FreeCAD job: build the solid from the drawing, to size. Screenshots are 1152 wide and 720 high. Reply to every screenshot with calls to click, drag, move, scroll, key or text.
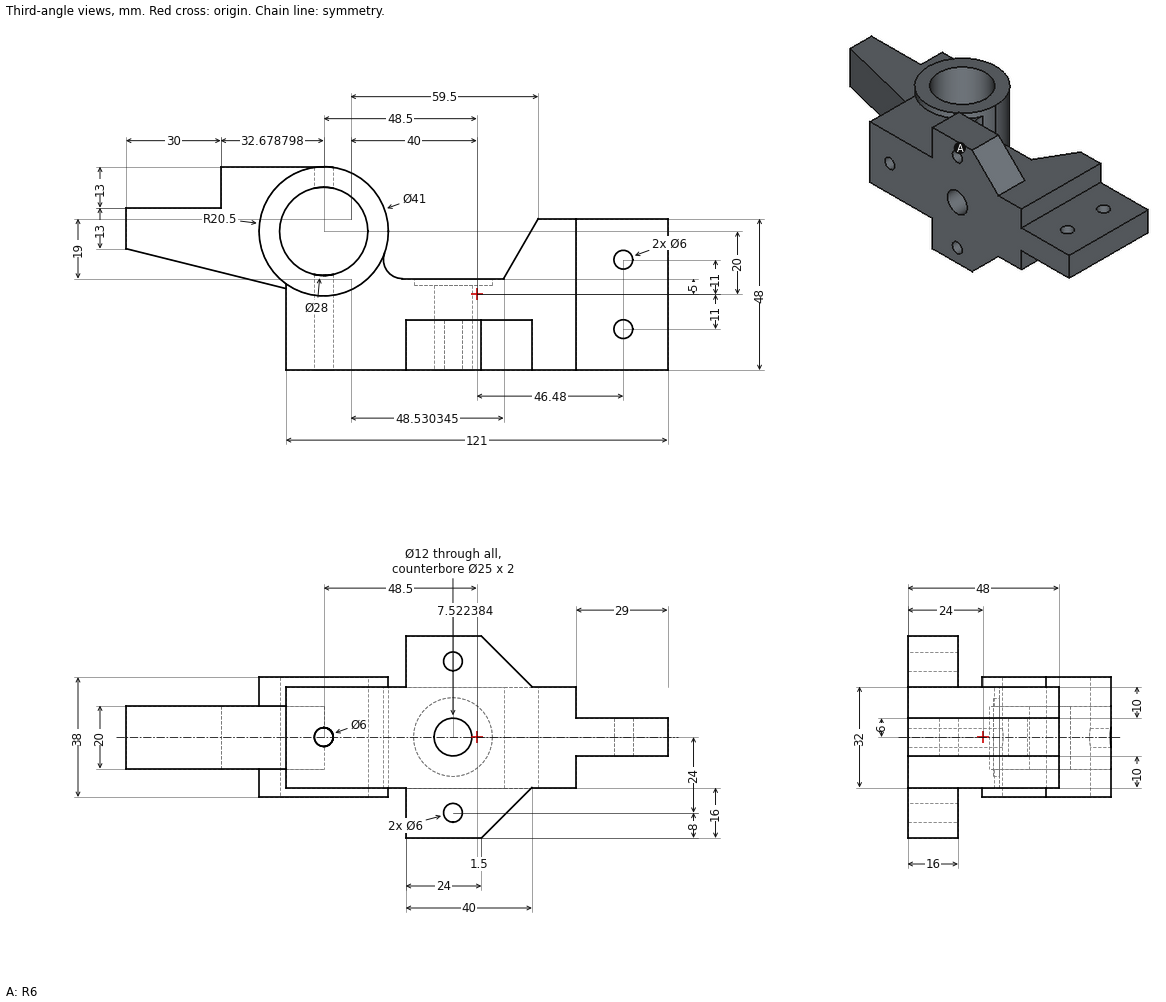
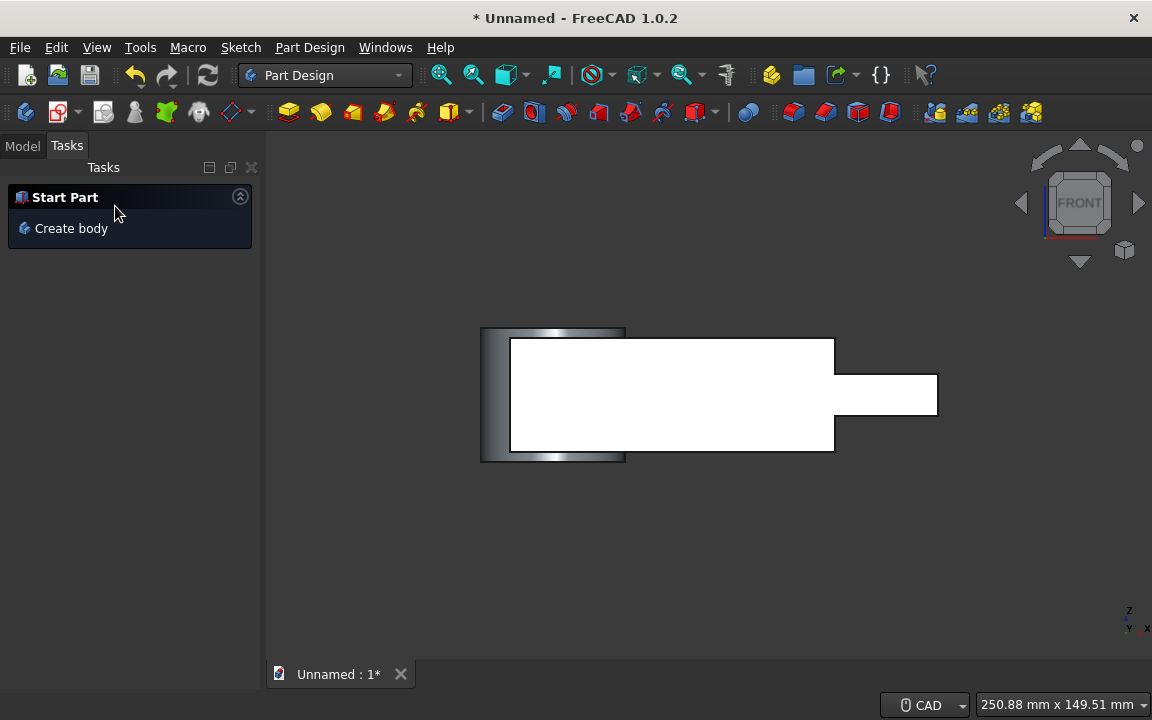
key(3)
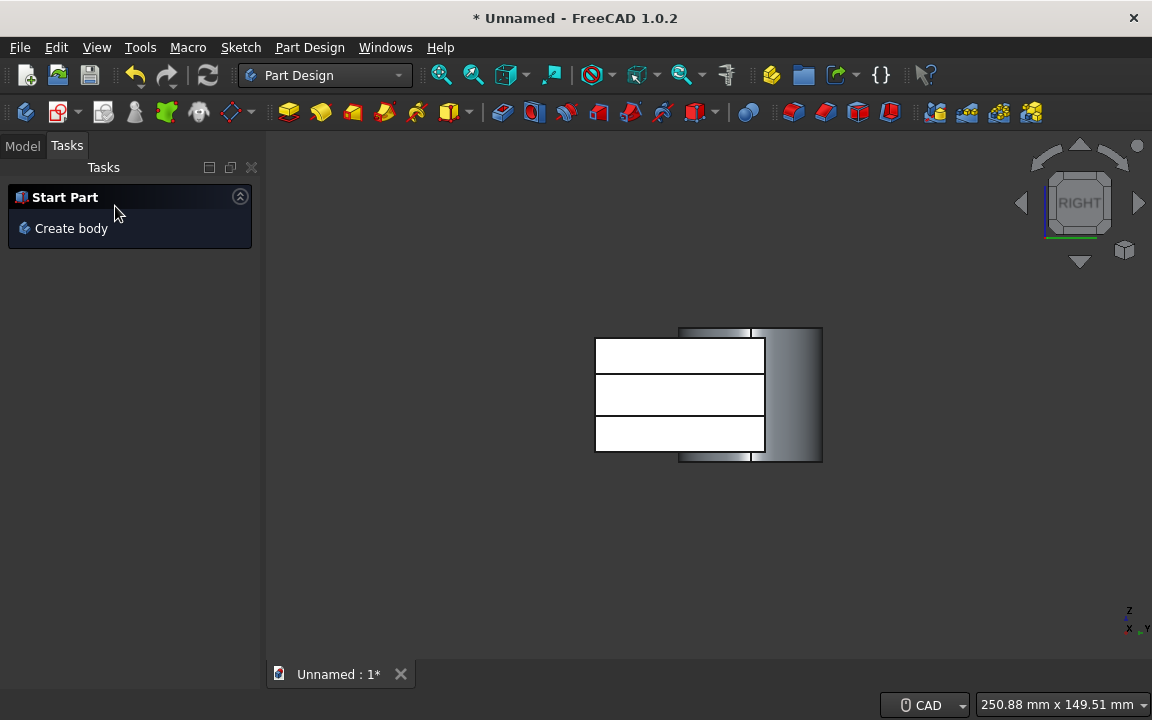
key(v)
key(f)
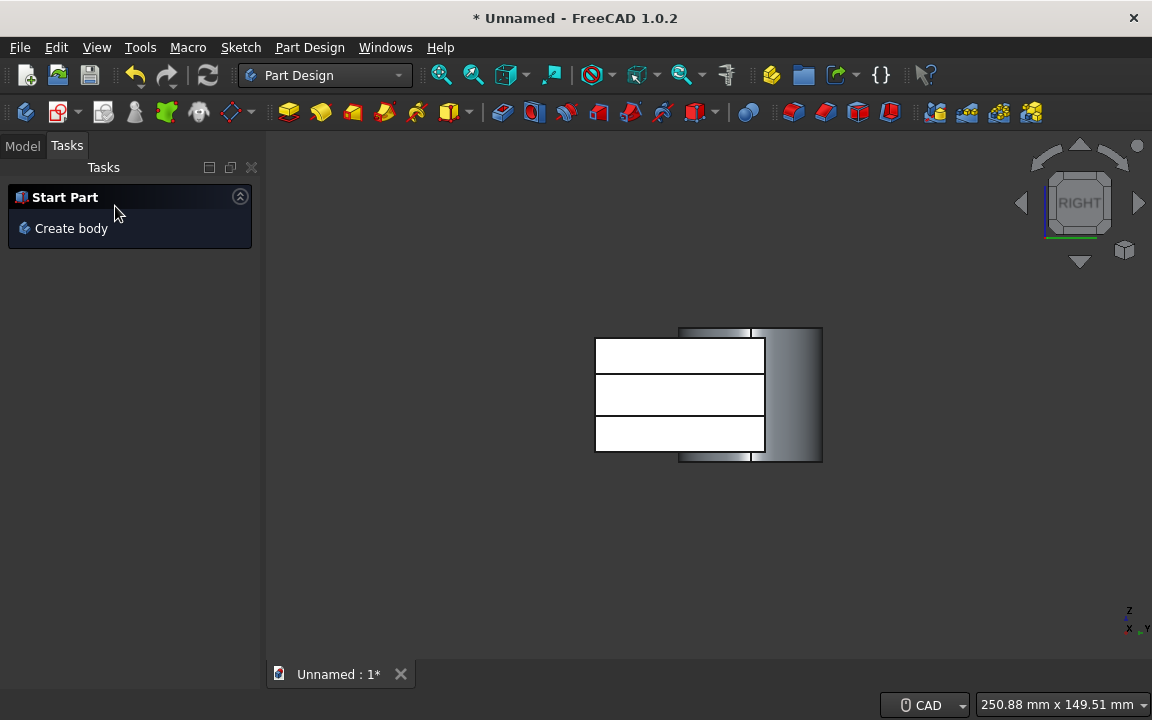
key(5)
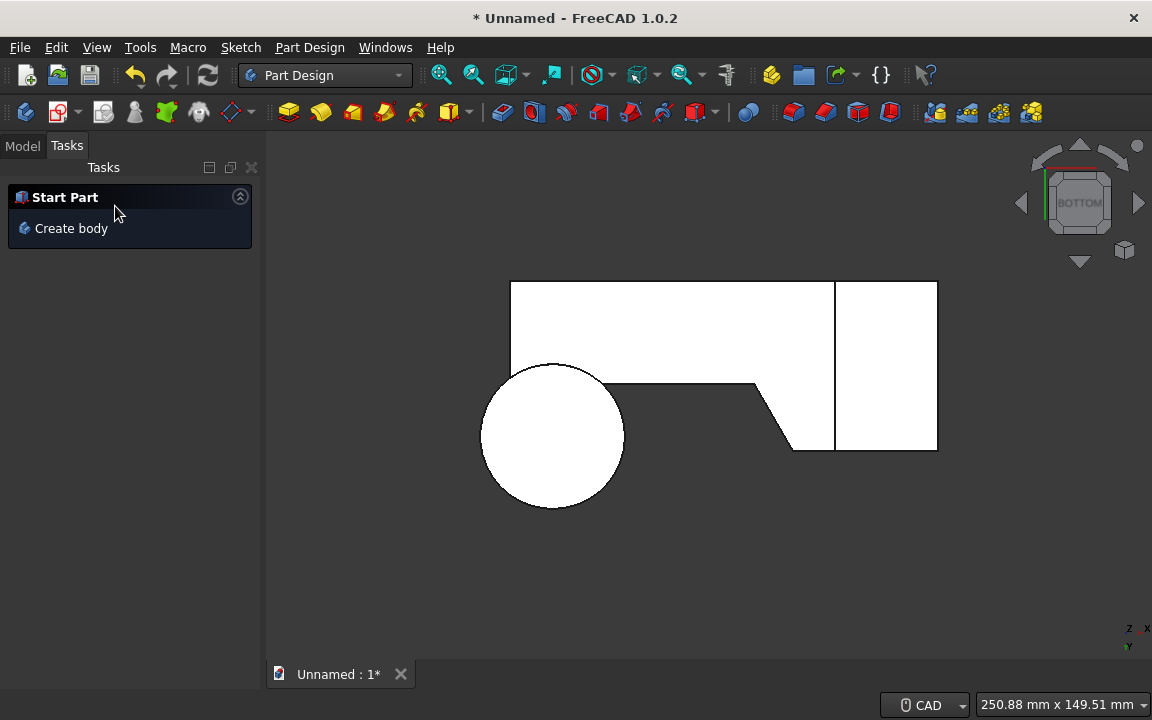
key(4)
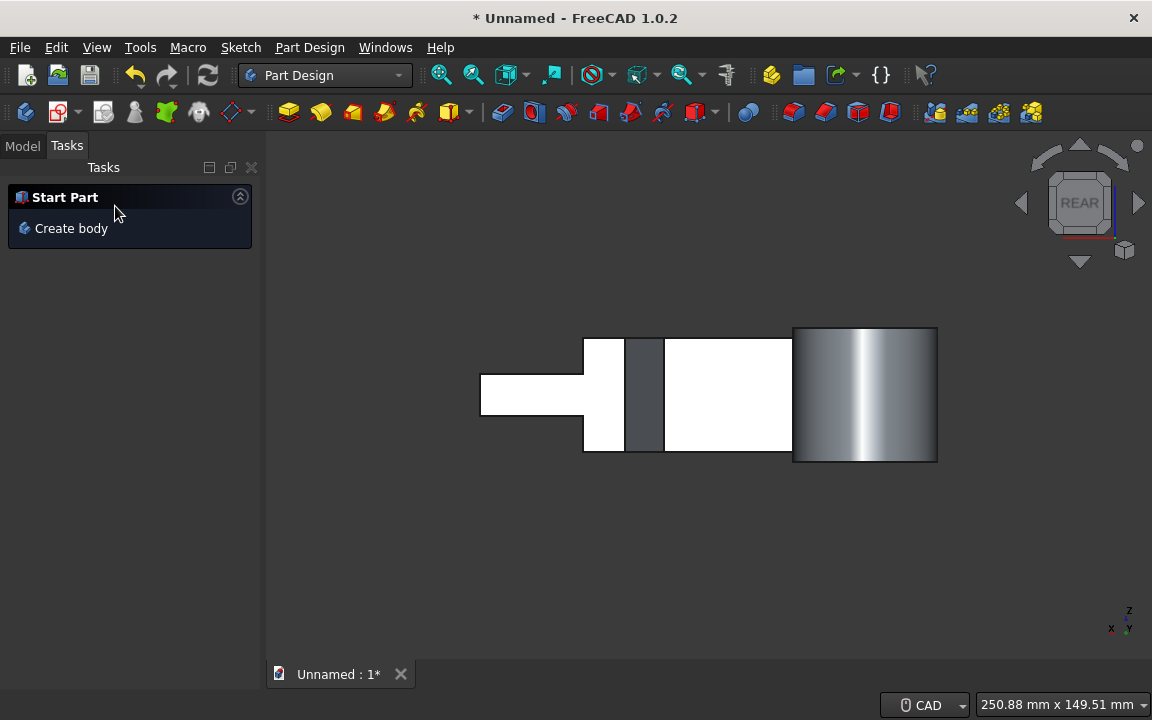
key(6)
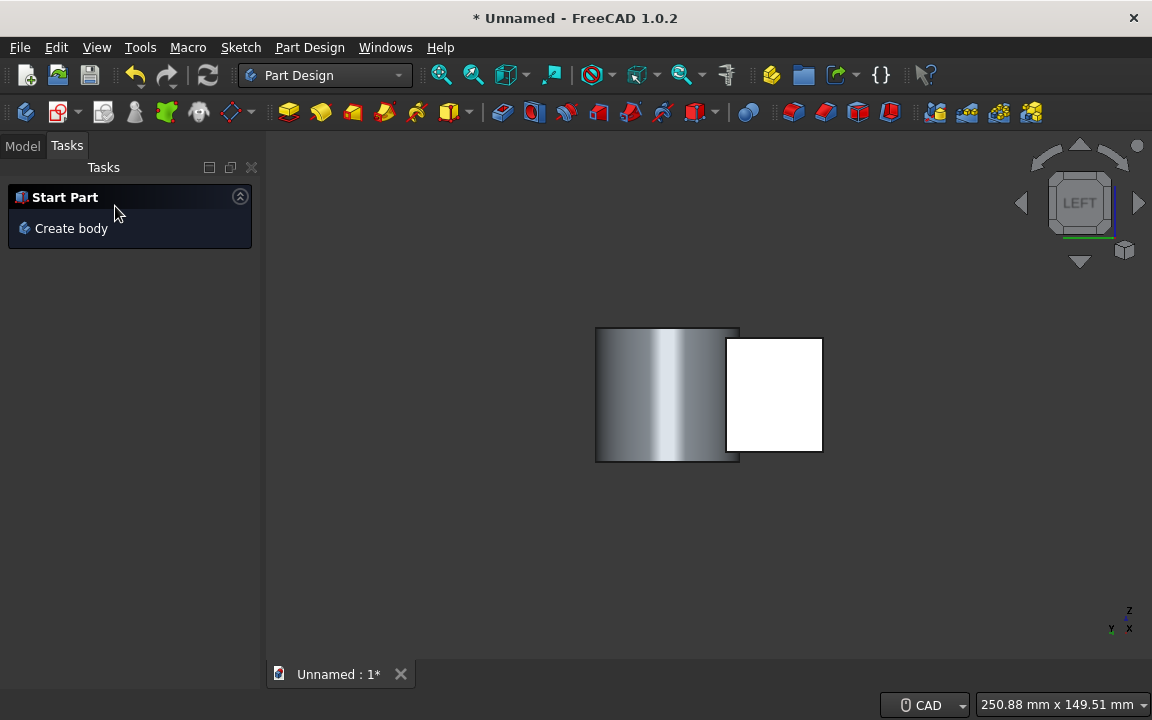
key(v)
key(f)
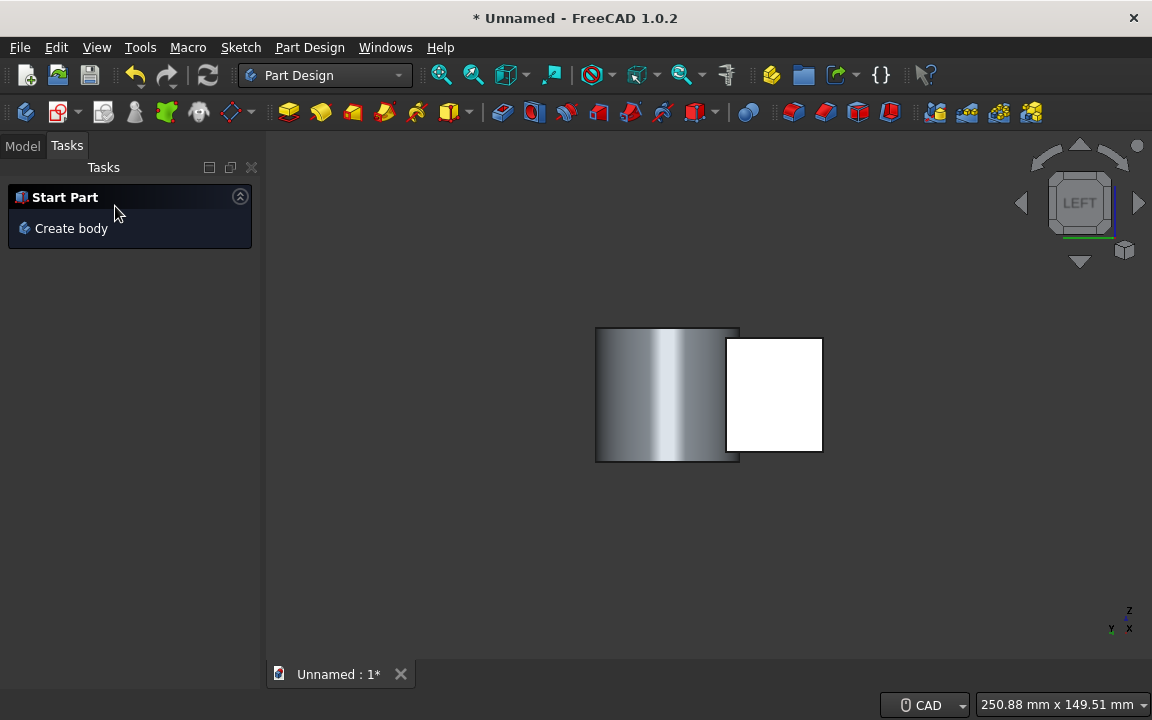
key(v)
key(3)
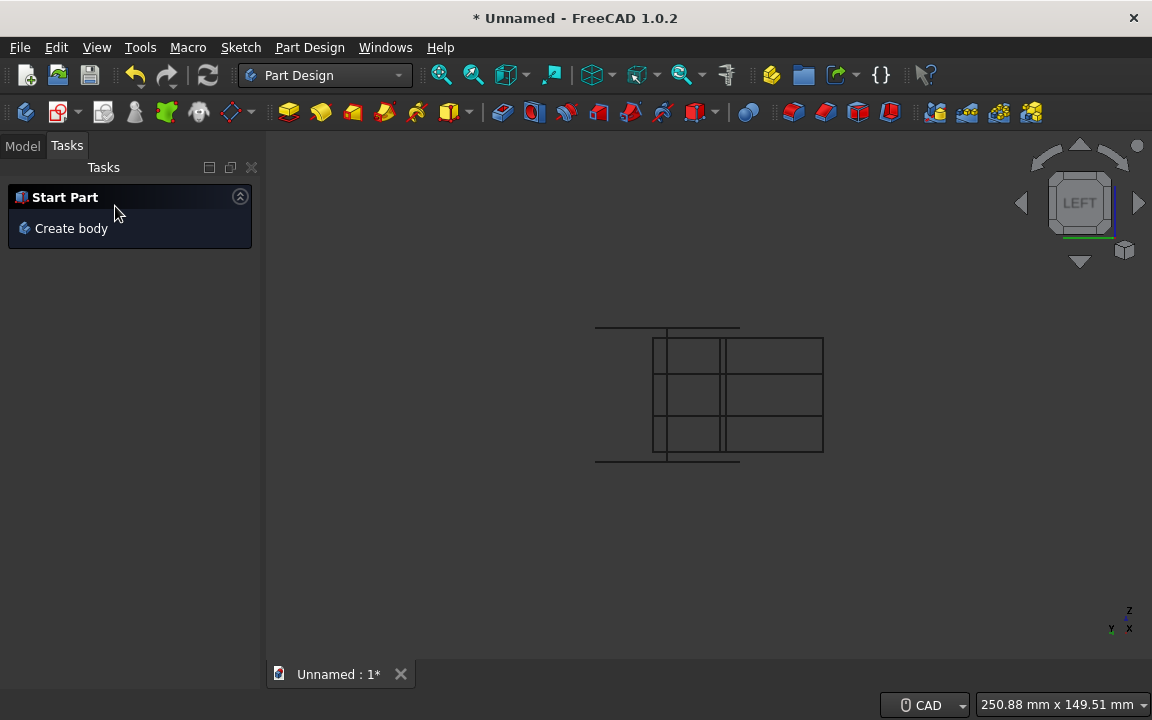
key(0)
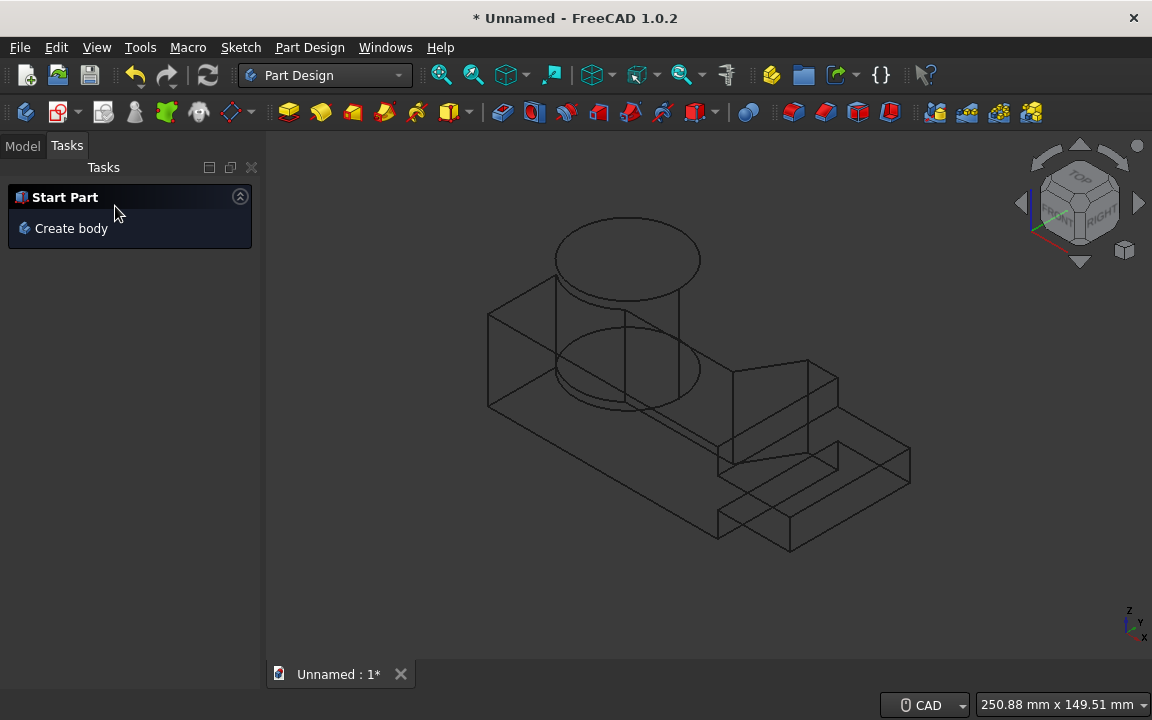
click(625, 355)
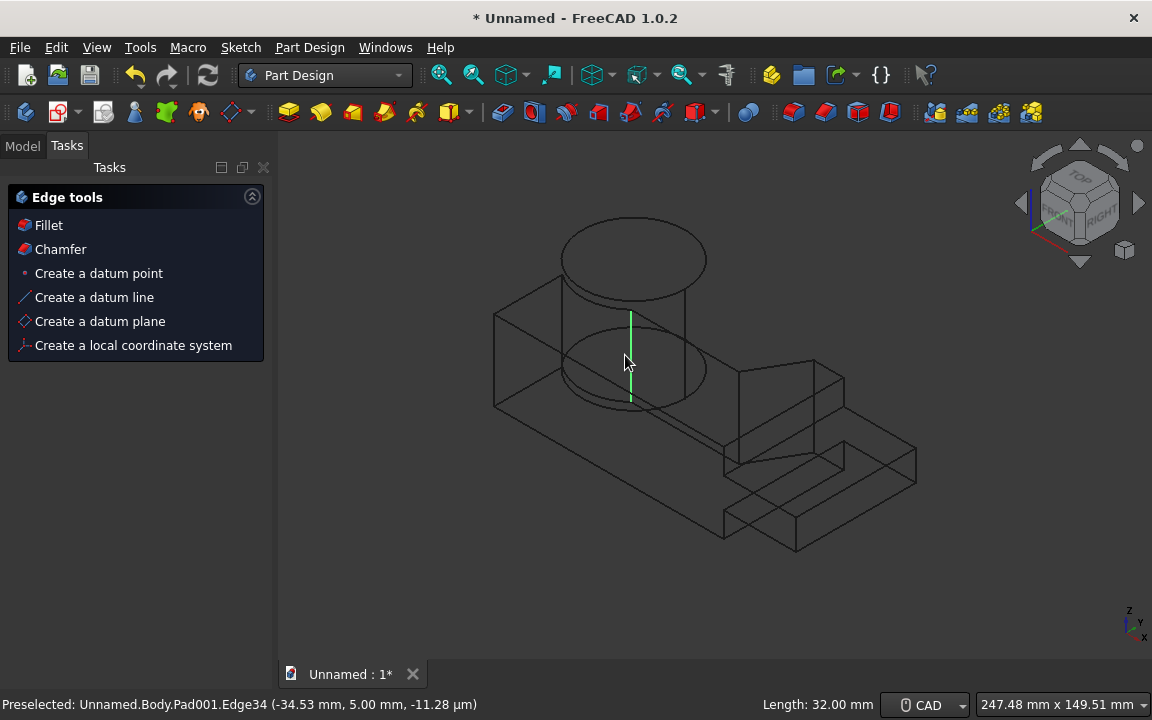
key(v)
key(1)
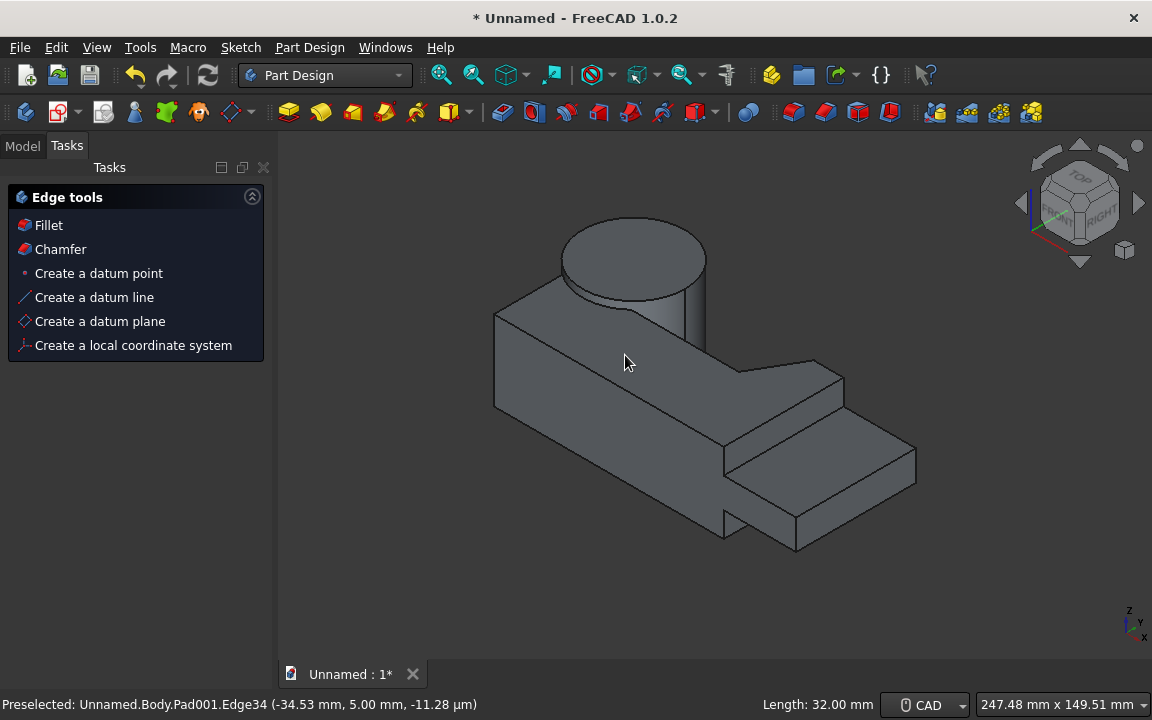
click(794, 112)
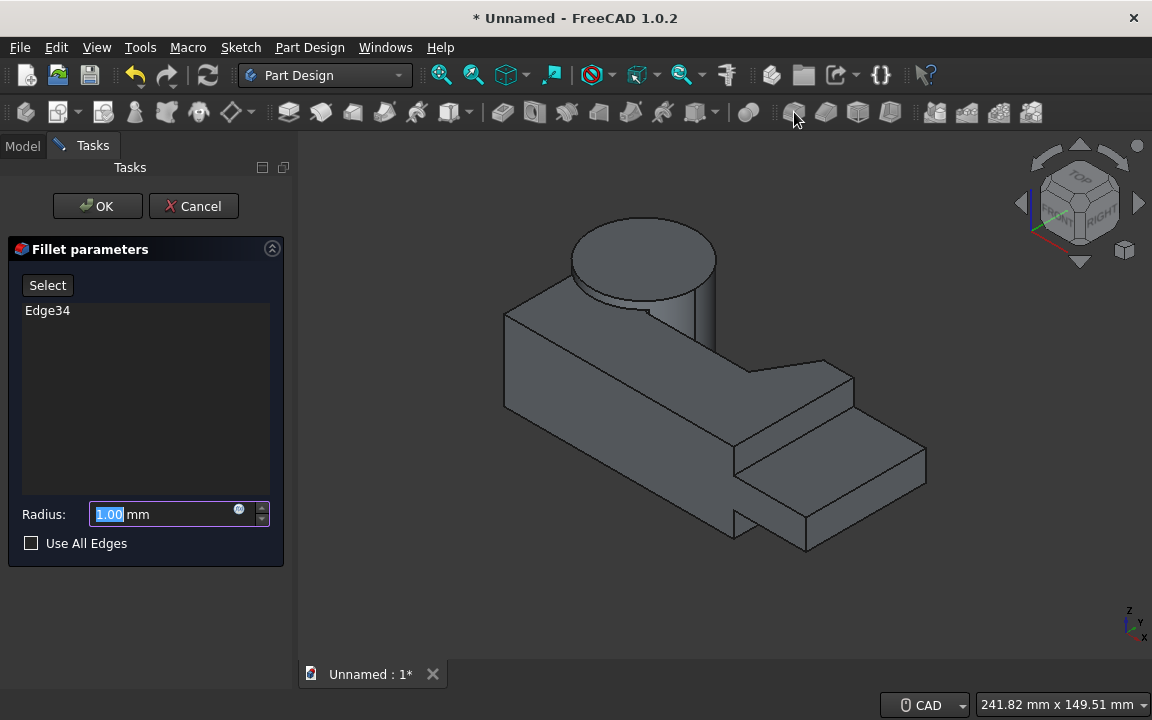
text(6)
key(Tab)